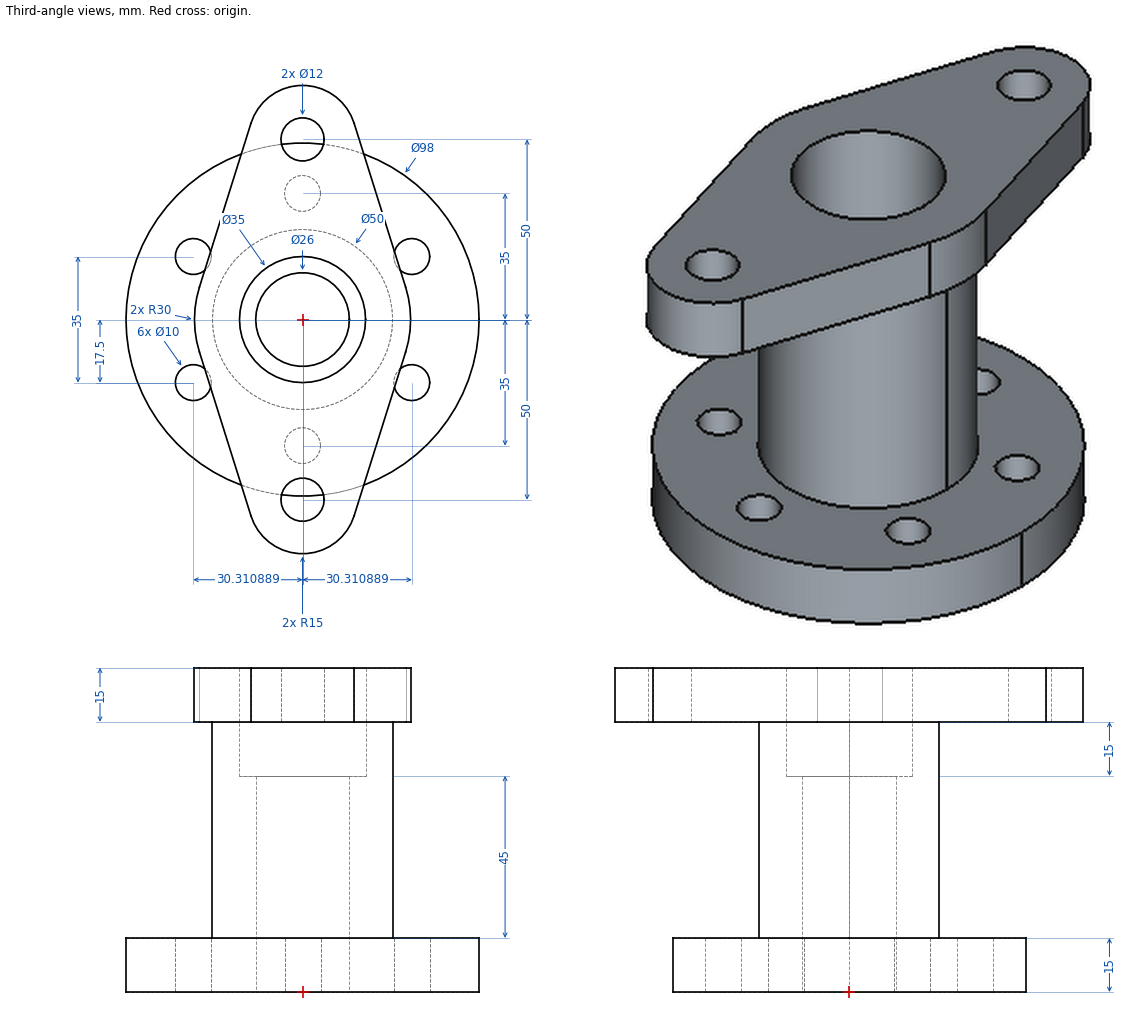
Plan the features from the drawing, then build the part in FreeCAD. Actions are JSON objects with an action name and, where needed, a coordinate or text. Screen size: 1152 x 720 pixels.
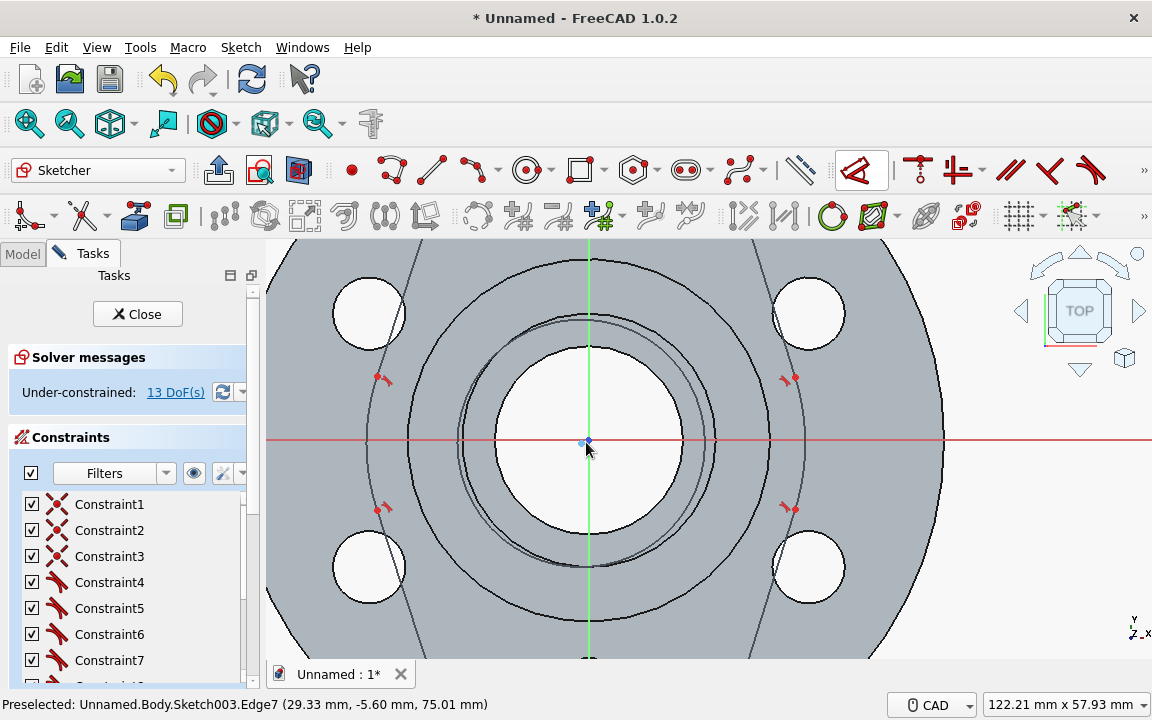
{"action": "left_click_drag", "start_coordinate": [571, 430], "coordinate": [599, 453]}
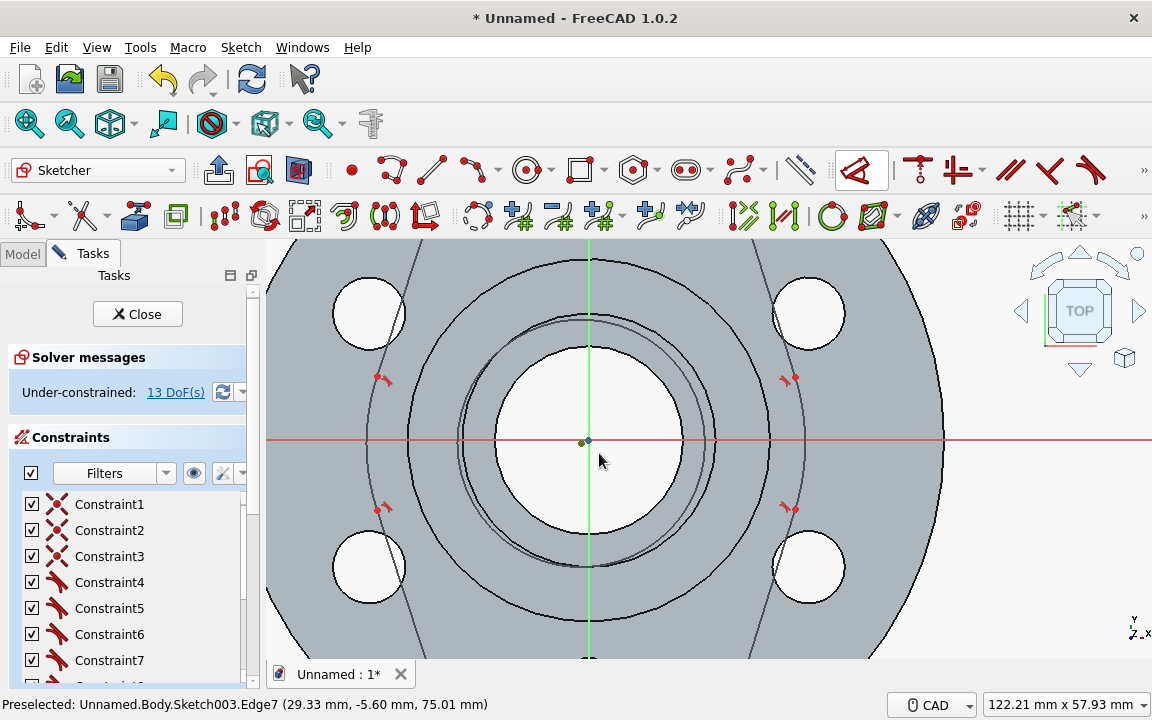
{"action": "key", "text": "c"}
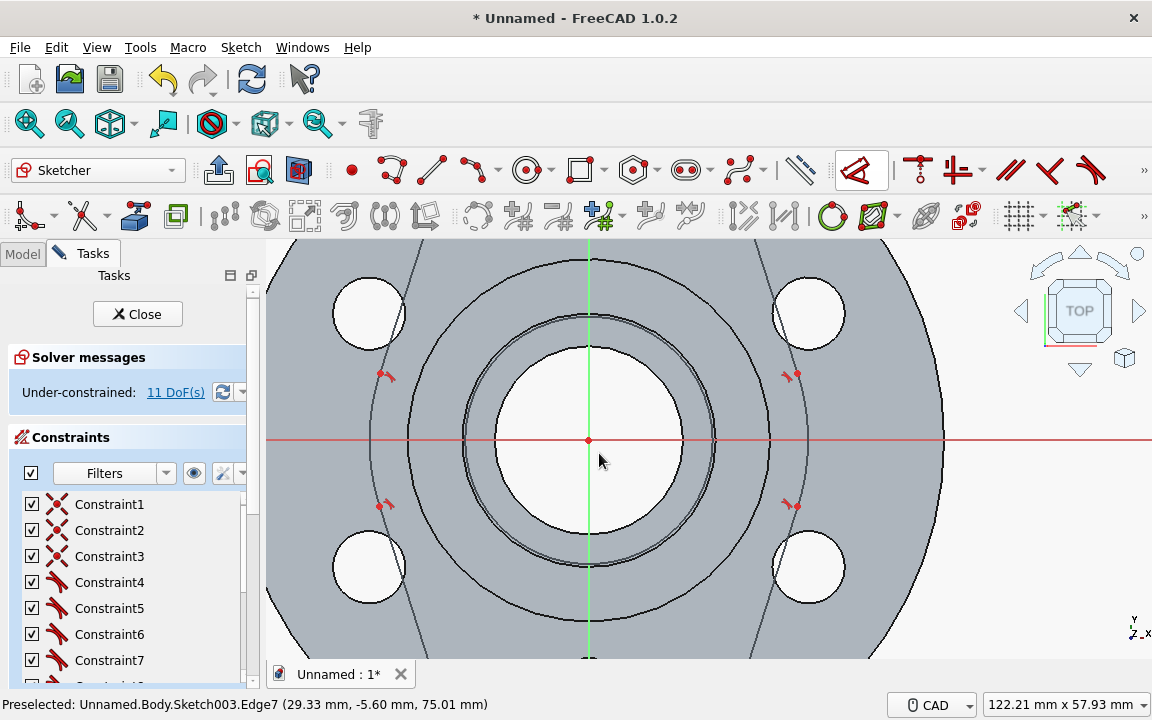
{"action": "left_click", "coordinate": [371, 413]}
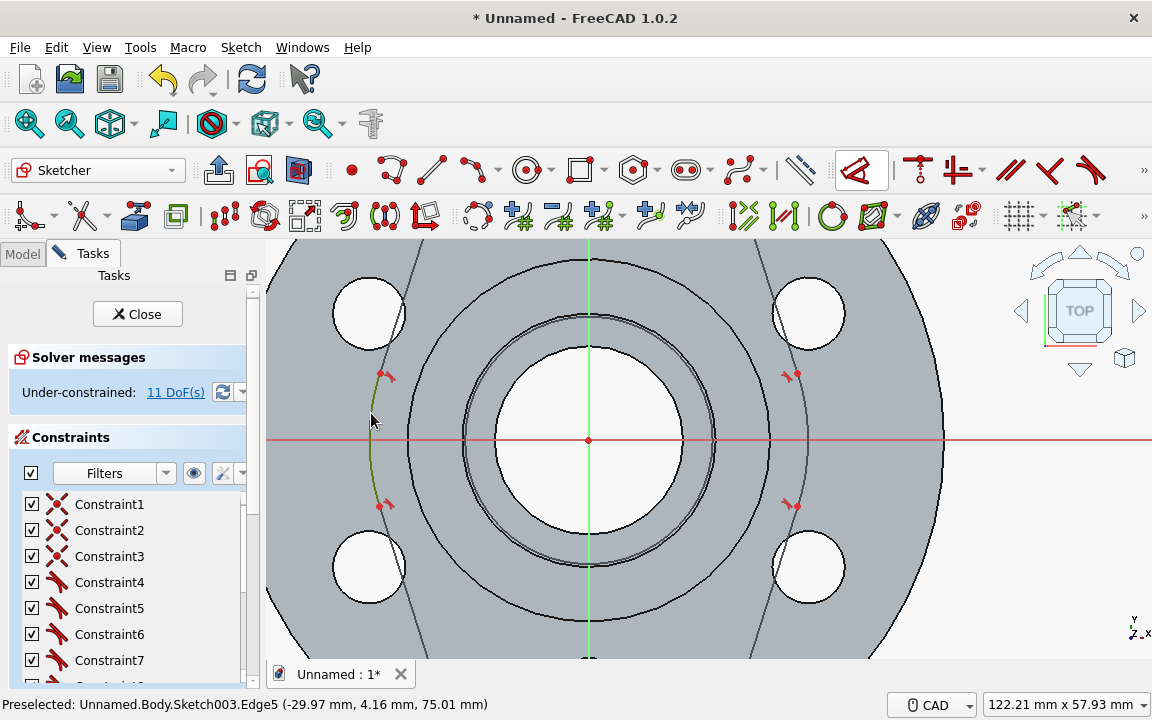
{"action": "left_click", "coordinate": [806, 467]}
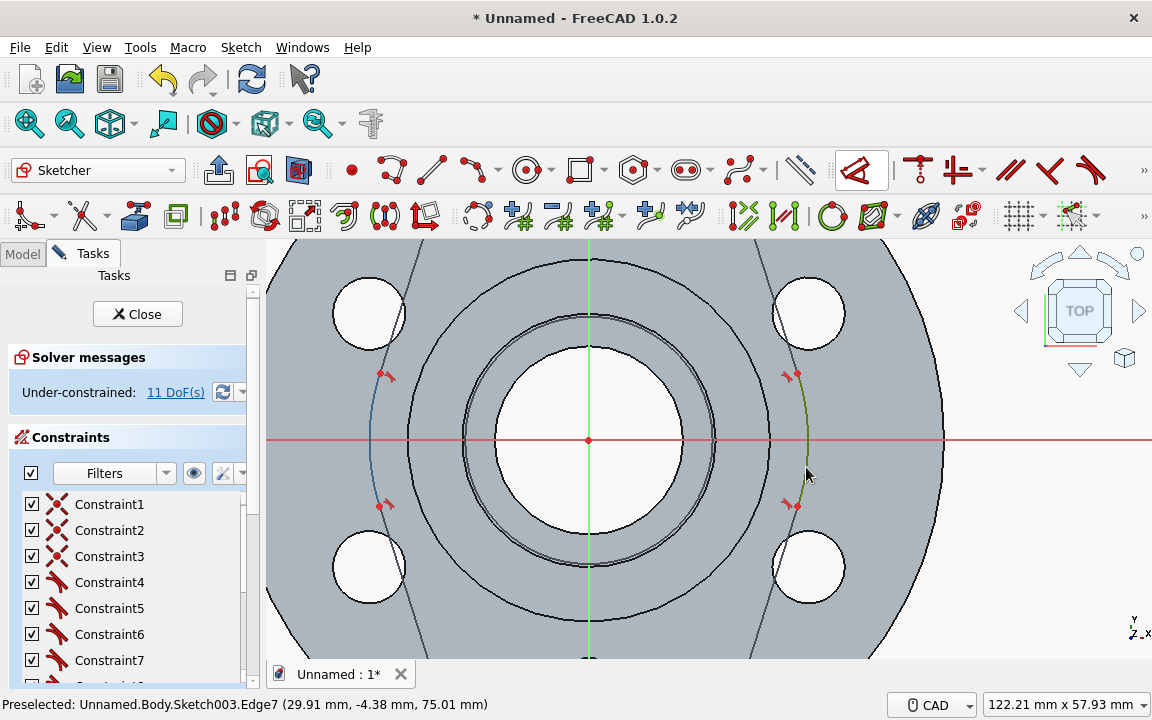
{"action": "key", "text": "e"}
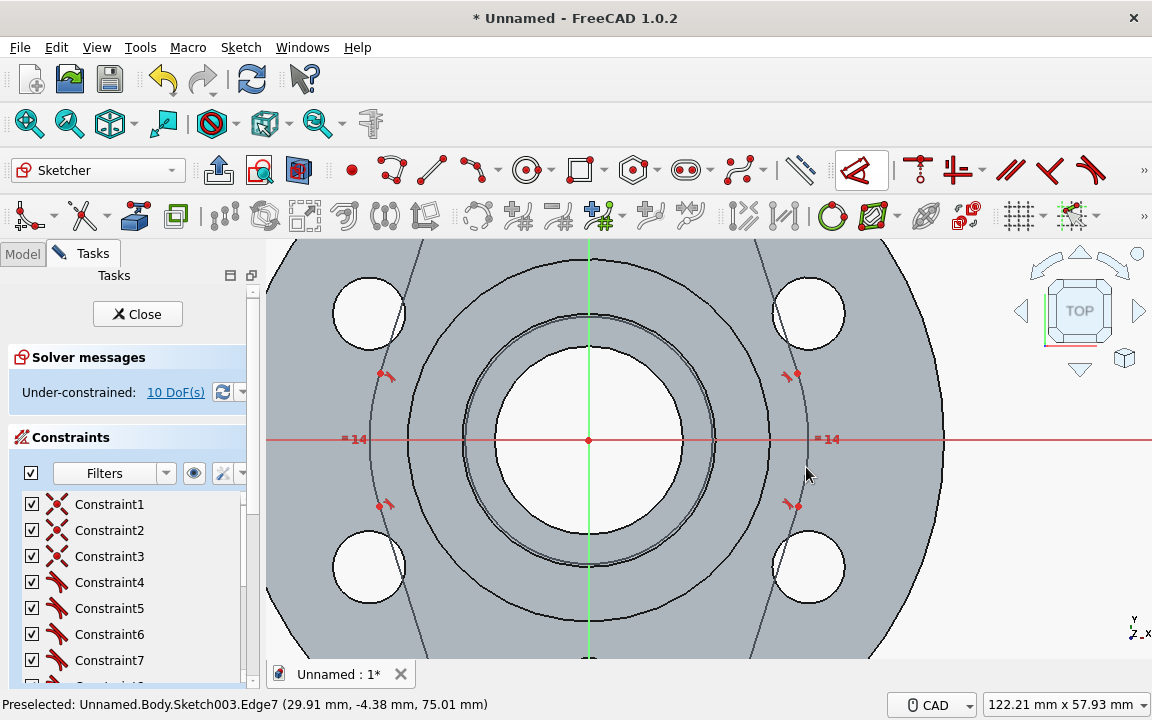
{"action": "scroll", "coordinate": [663, 453], "scroll_direction": "down", "scroll_amount": 6}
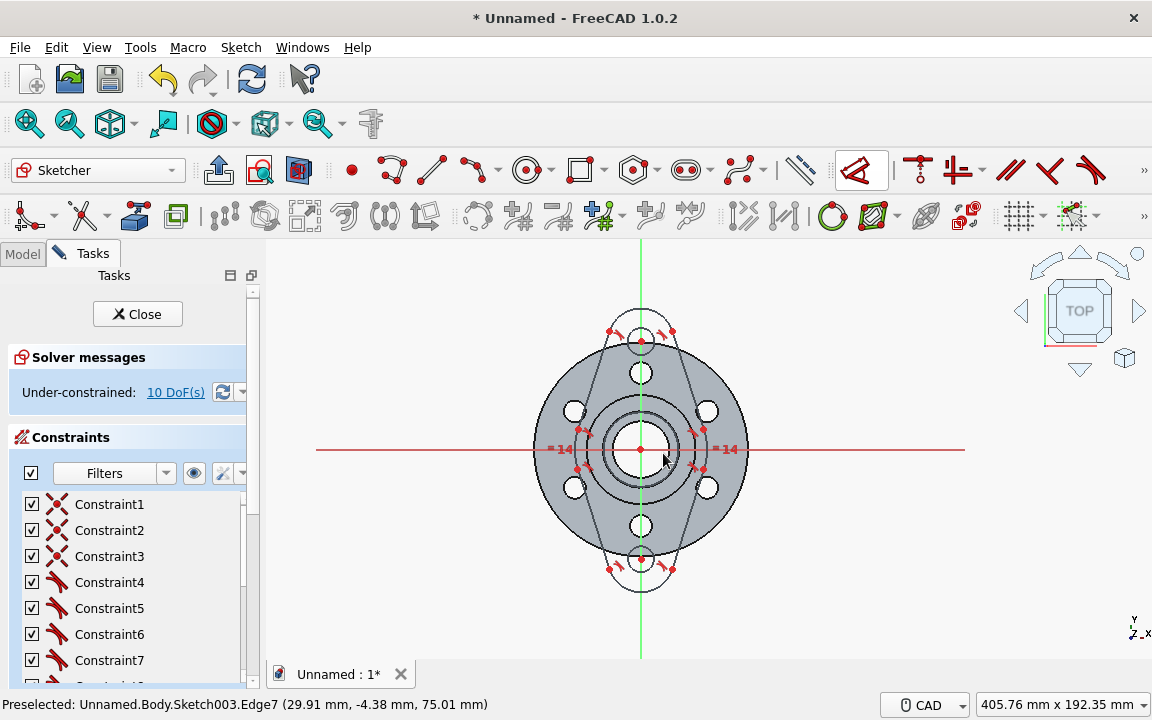
{"action": "left_click", "coordinate": [625, 588]}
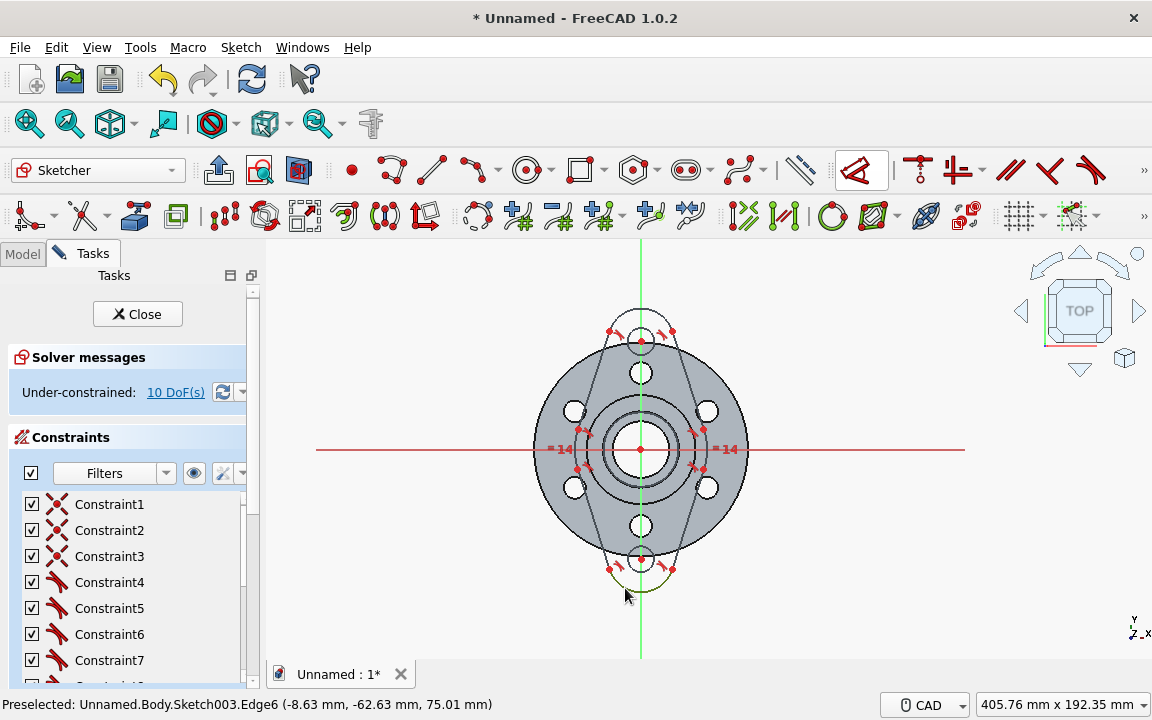
{"action": "left_click", "coordinate": [657, 313]}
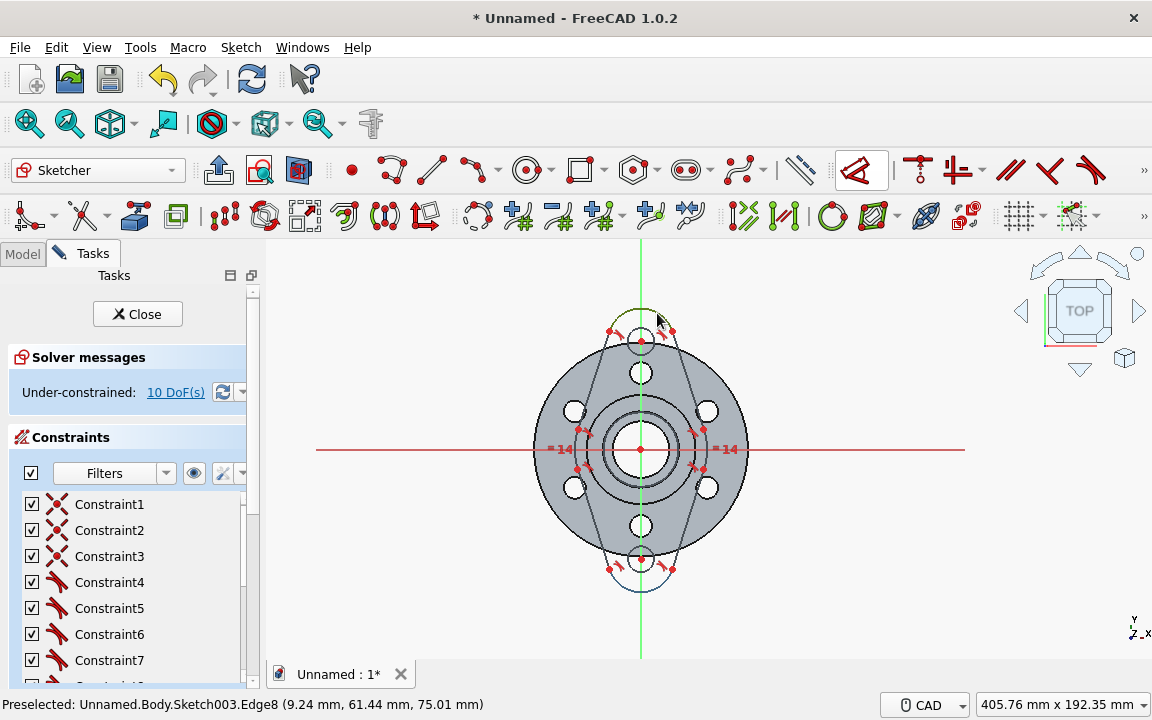
{"action": "key", "text": "e"}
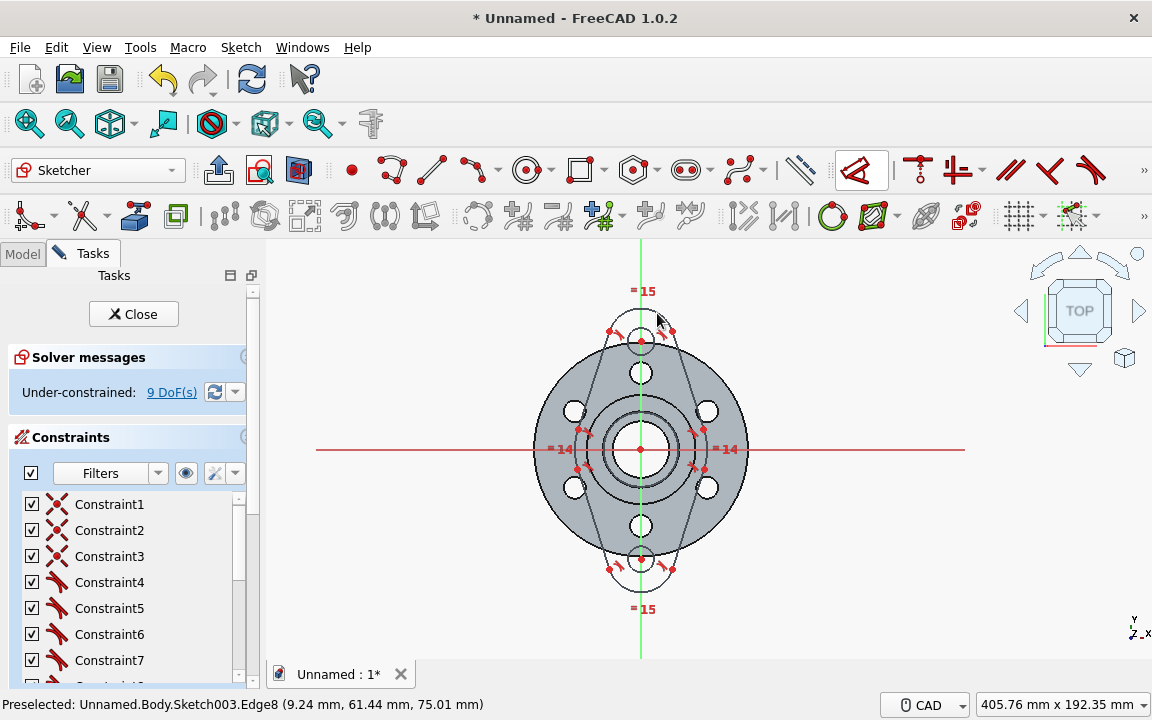
{"action": "scroll", "coordinate": [650, 332], "scroll_direction": "up", "scroll_amount": 2}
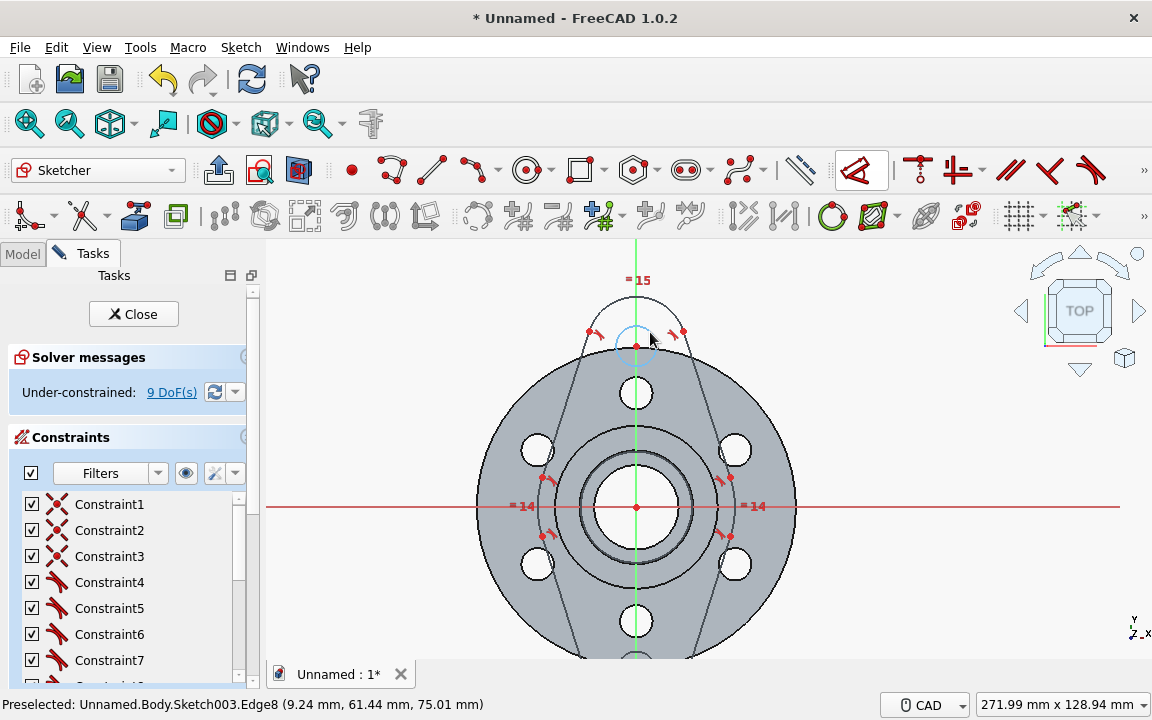
{"action": "left_click", "coordinate": [651, 332]}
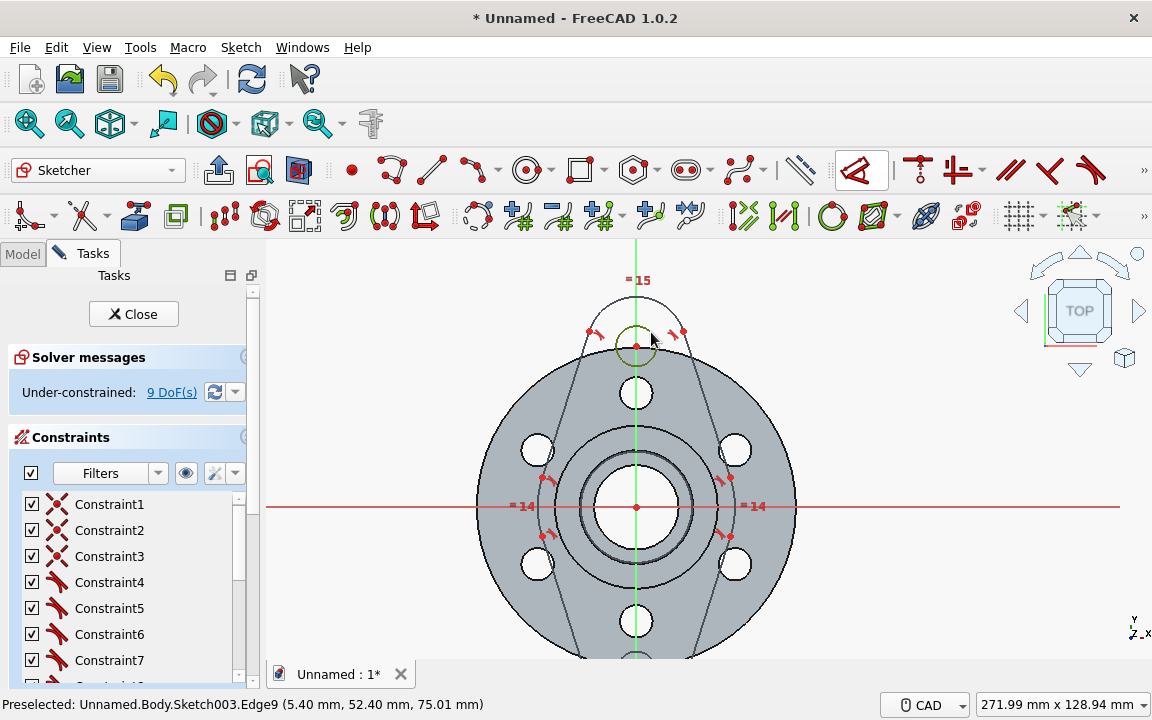
{"action": "scroll", "coordinate": [649, 331], "scroll_direction": "down", "scroll_amount": 2}